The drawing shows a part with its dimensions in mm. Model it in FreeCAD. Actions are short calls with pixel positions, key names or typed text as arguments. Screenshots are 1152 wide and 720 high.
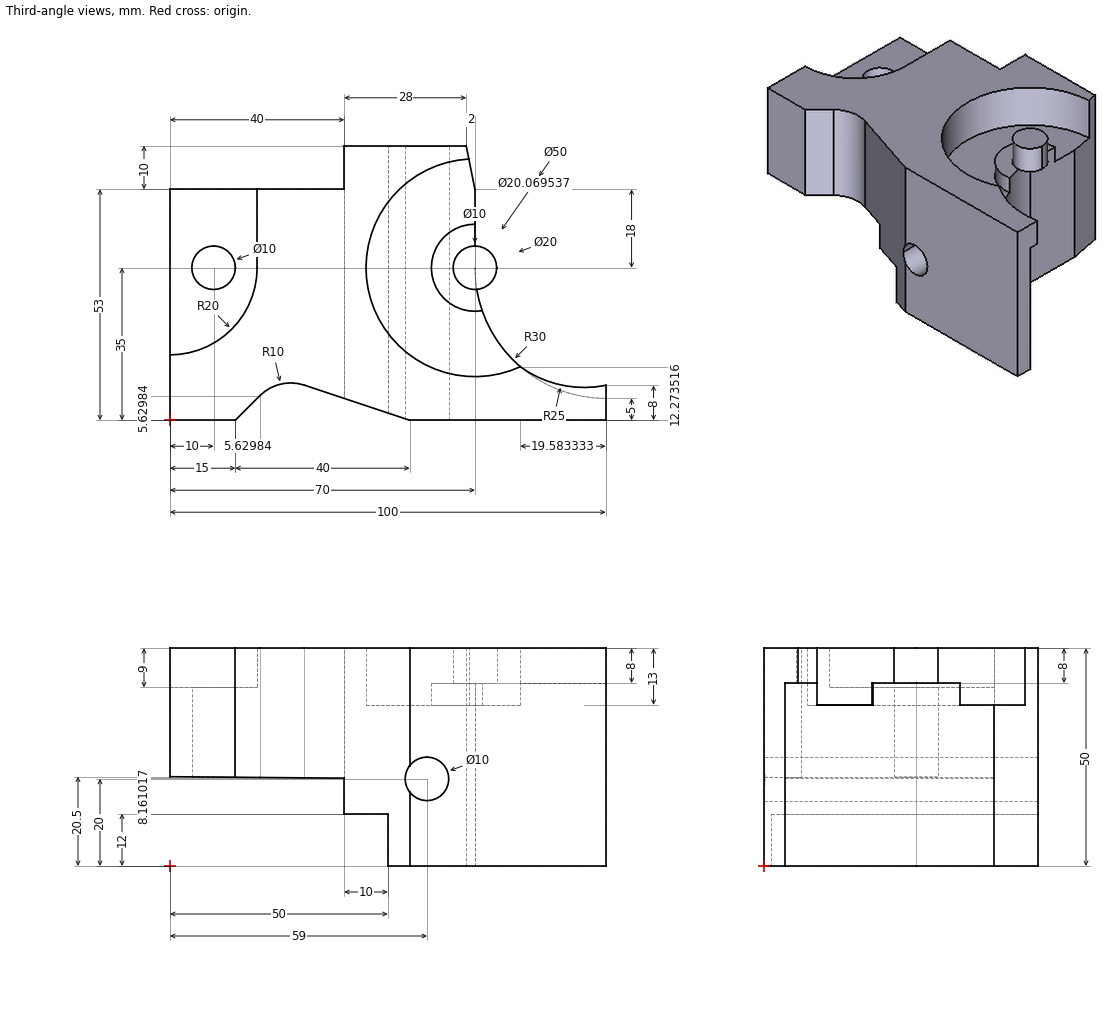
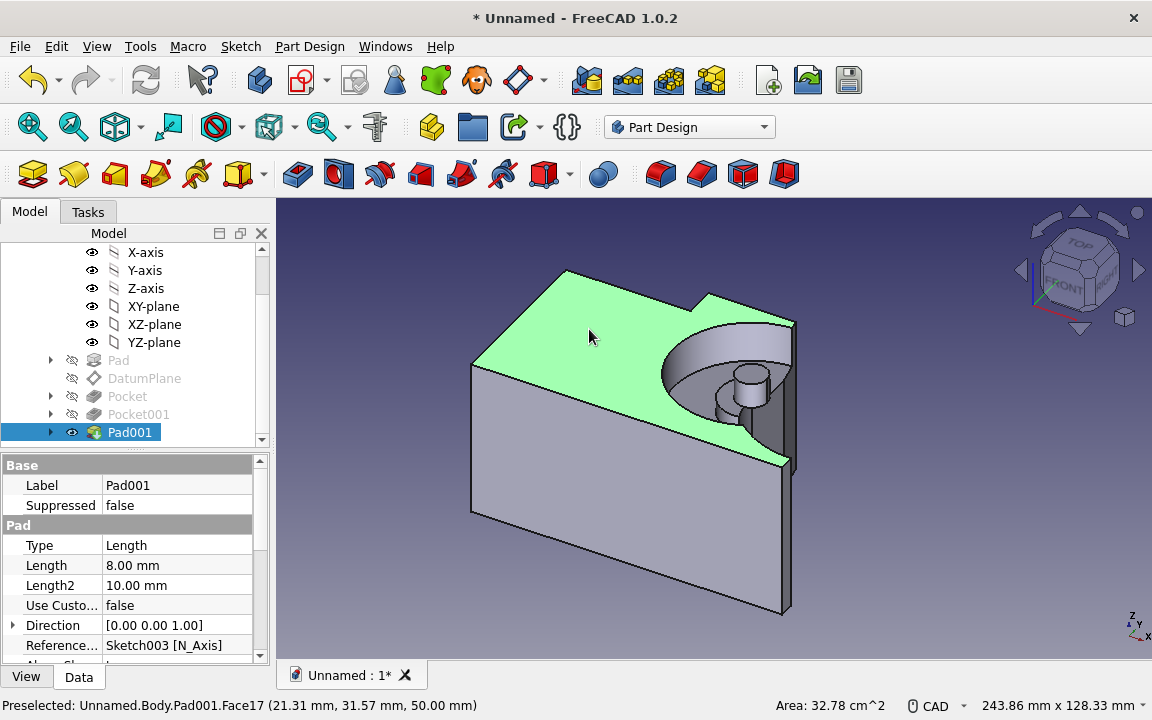
click(300, 80)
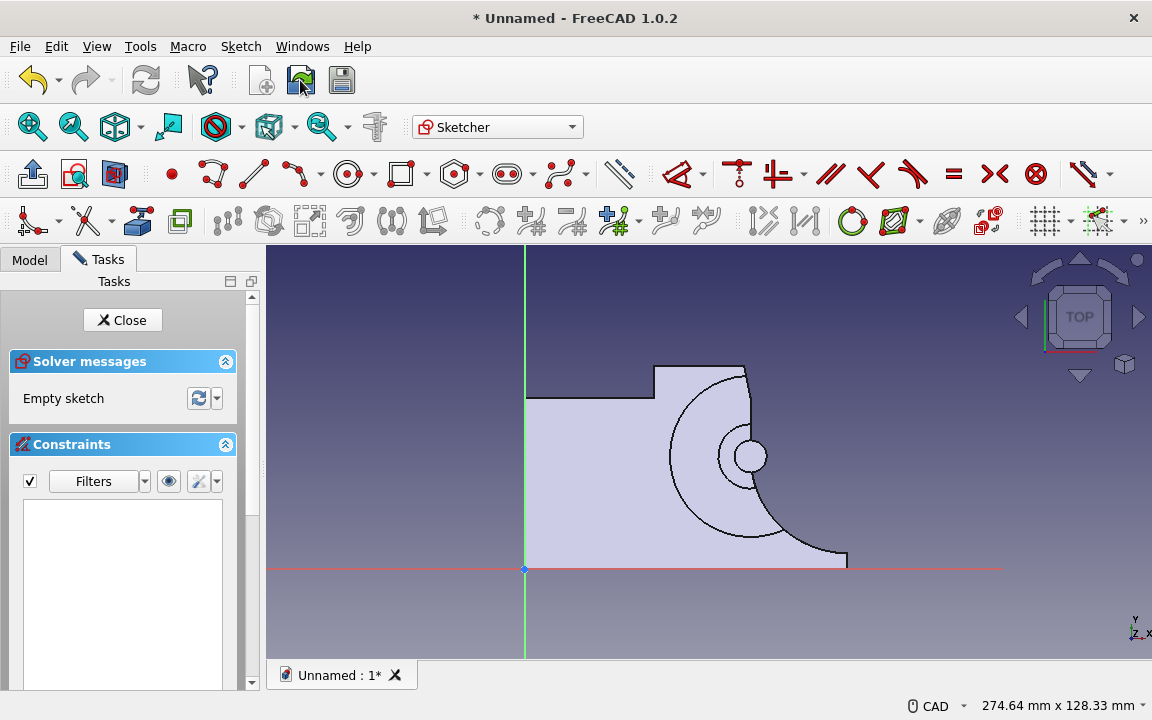
scroll(851, 569, up, 9)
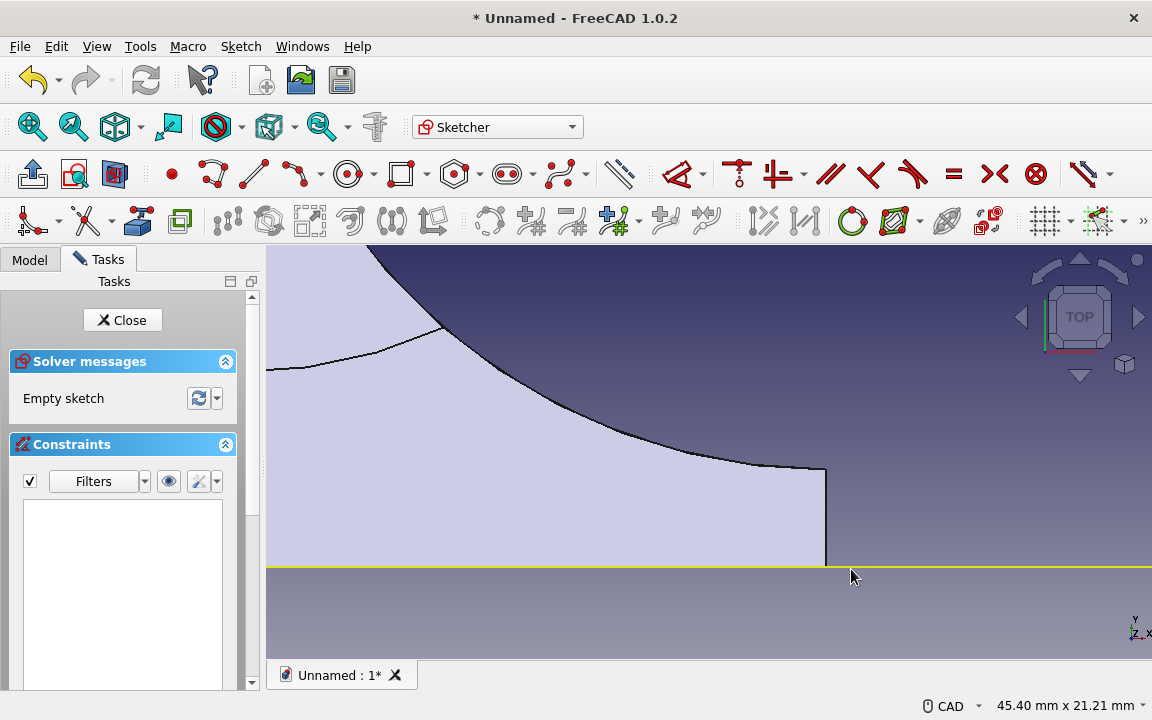
click(213, 174)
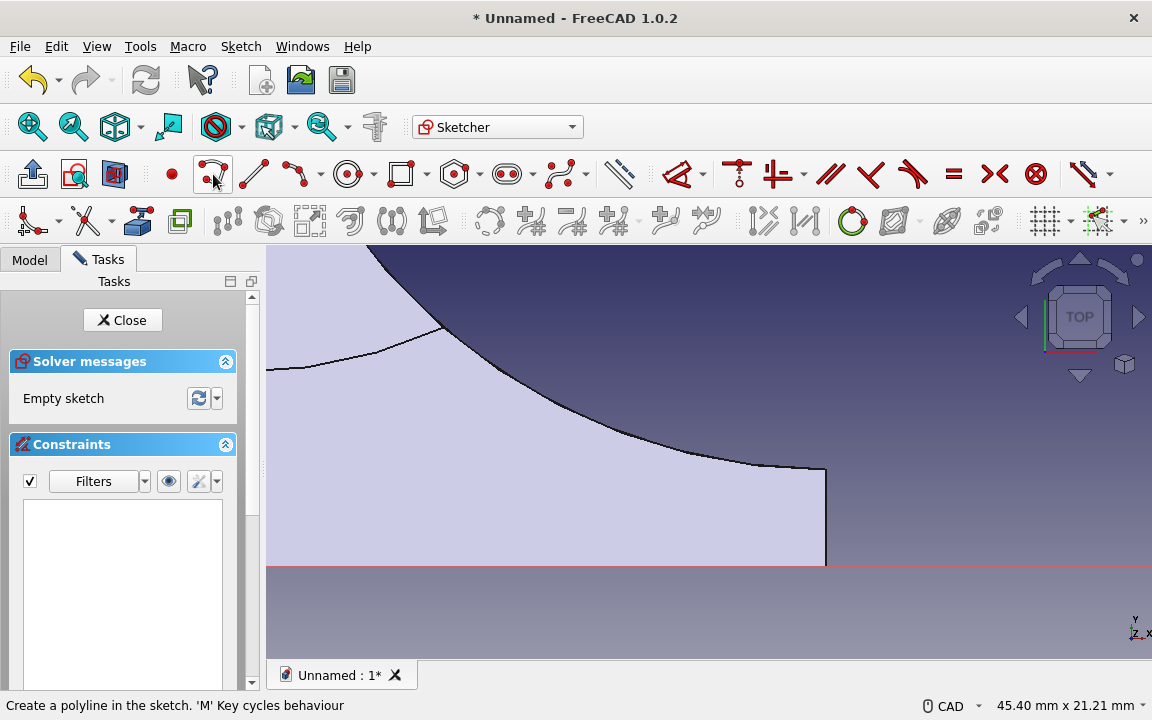
click(444, 328)
click(444, 567)
click(826, 558)
click(826, 411)
right_click(826, 411)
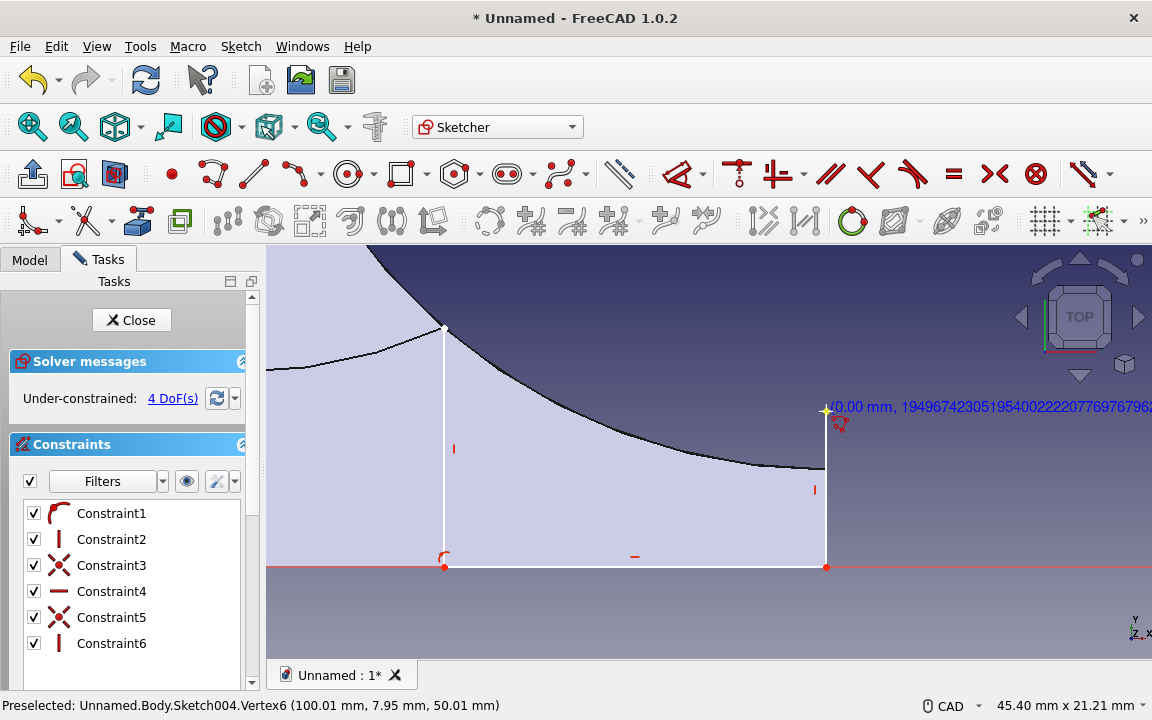
click(294, 174)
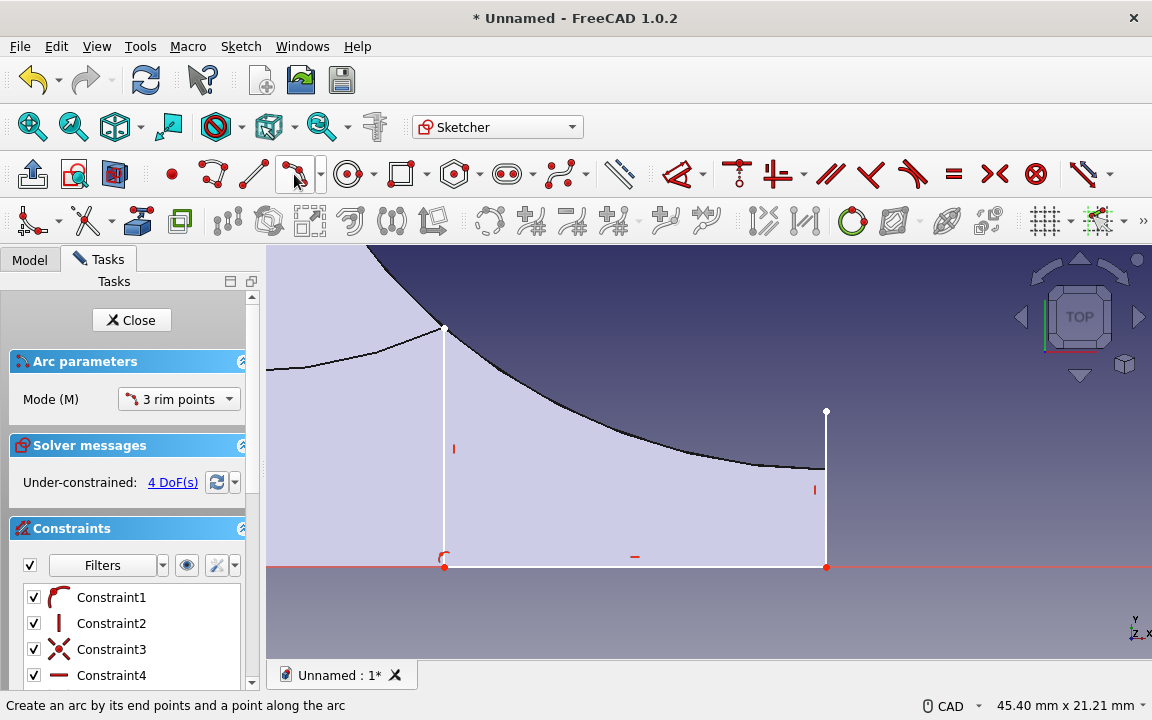
click(826, 412)
click(444, 329)
click(626, 409)
key(Escape)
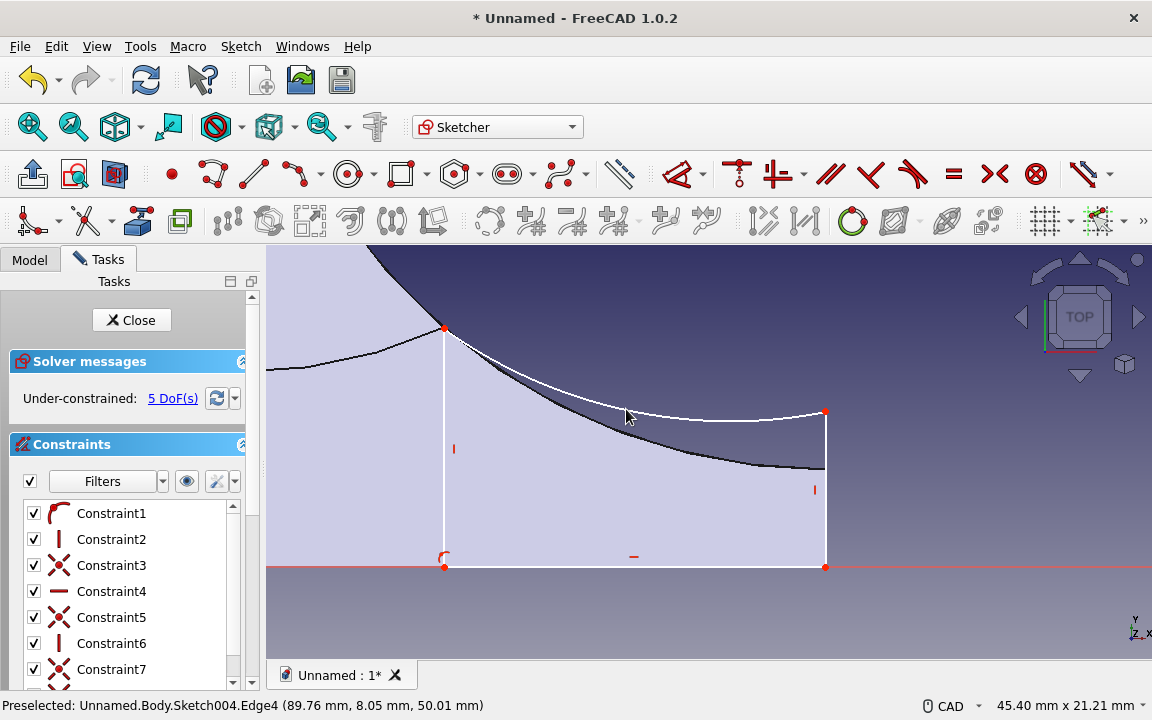
click(676, 174)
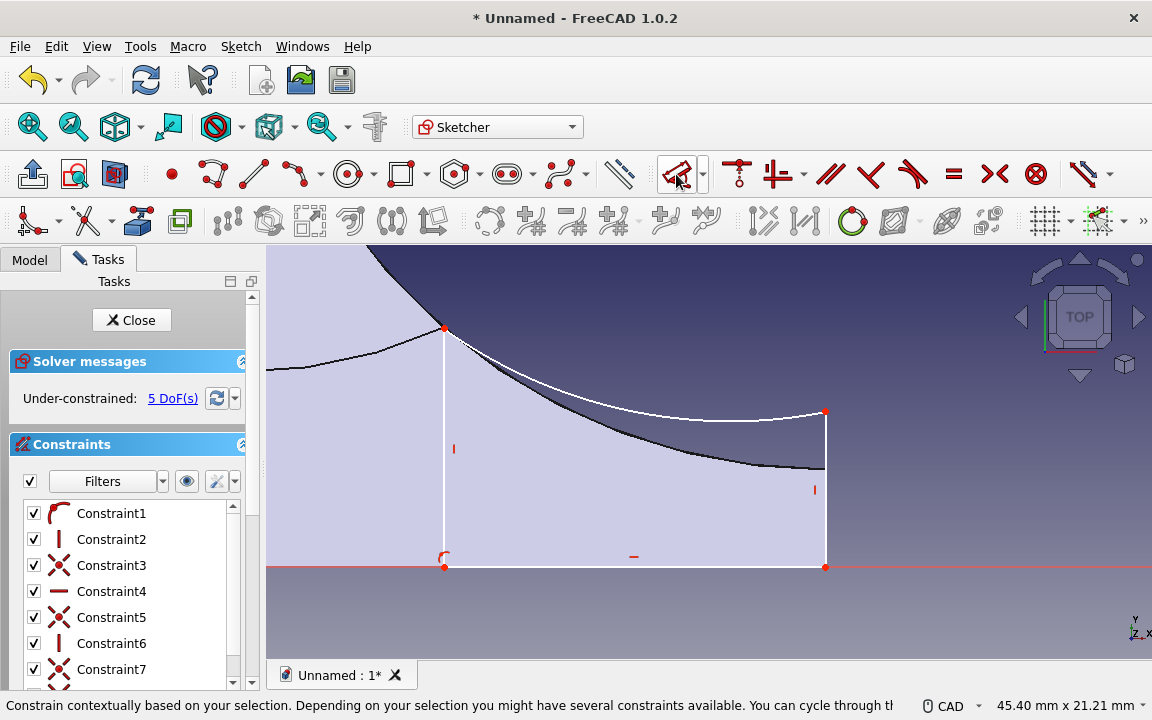
click(550, 387)
click(538, 417)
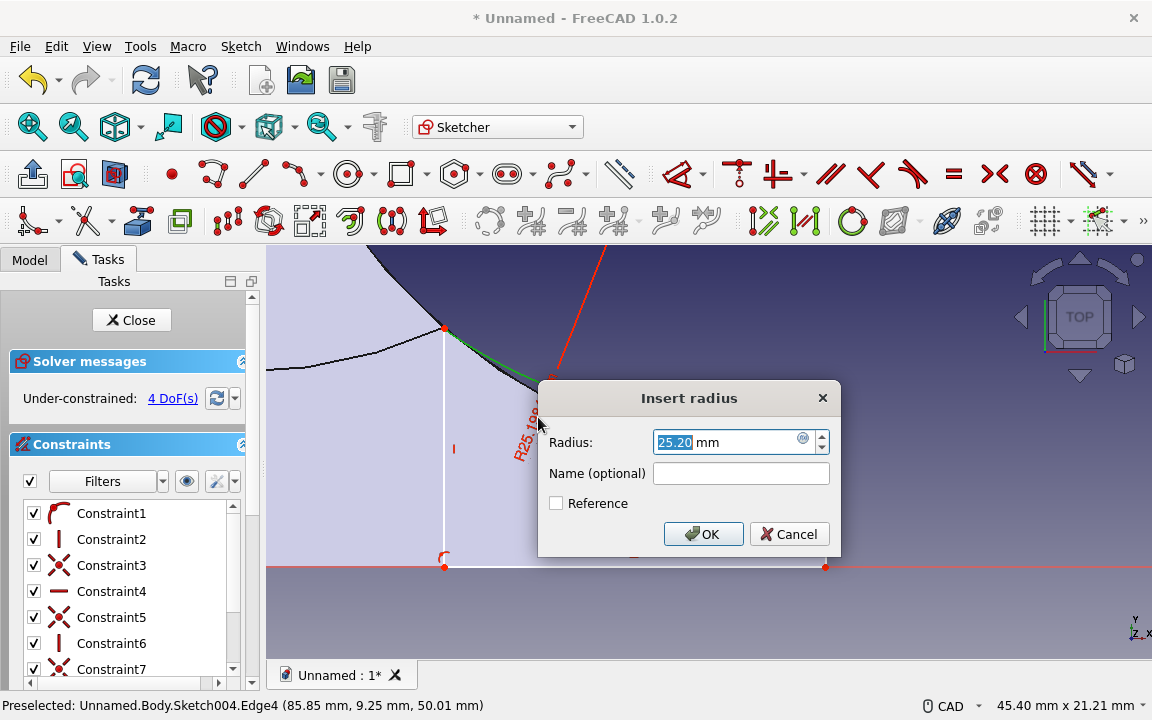
text(25)
key(Return)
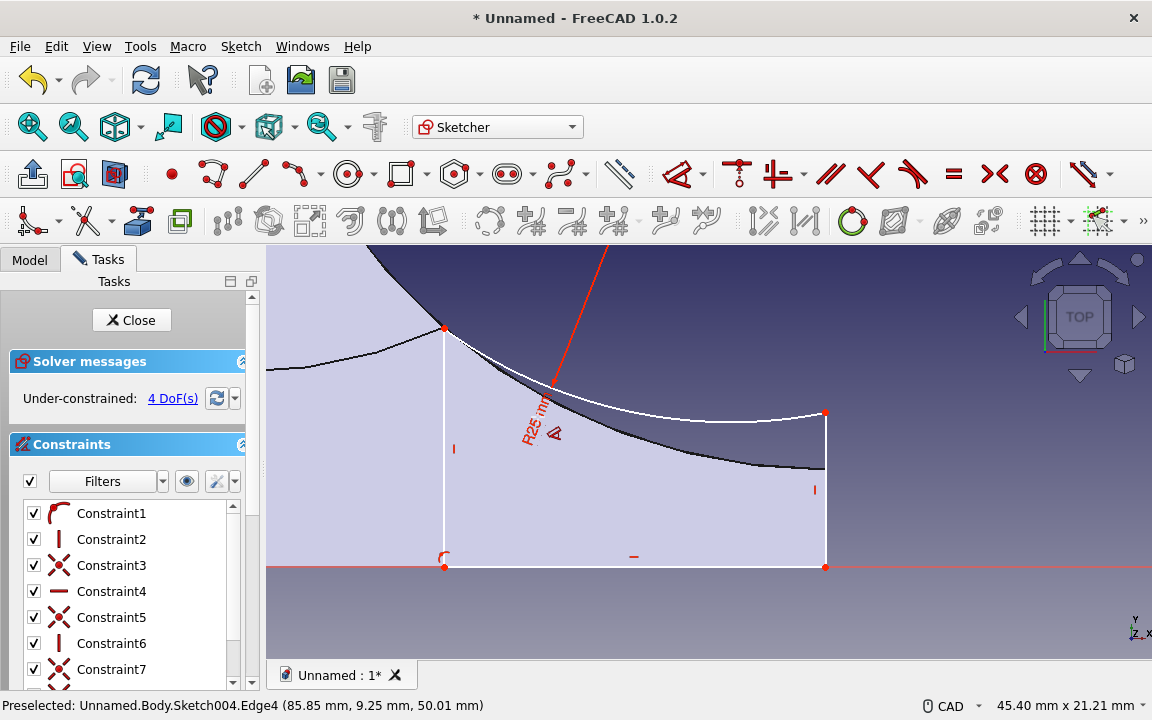
click(826, 521)
click(860, 490)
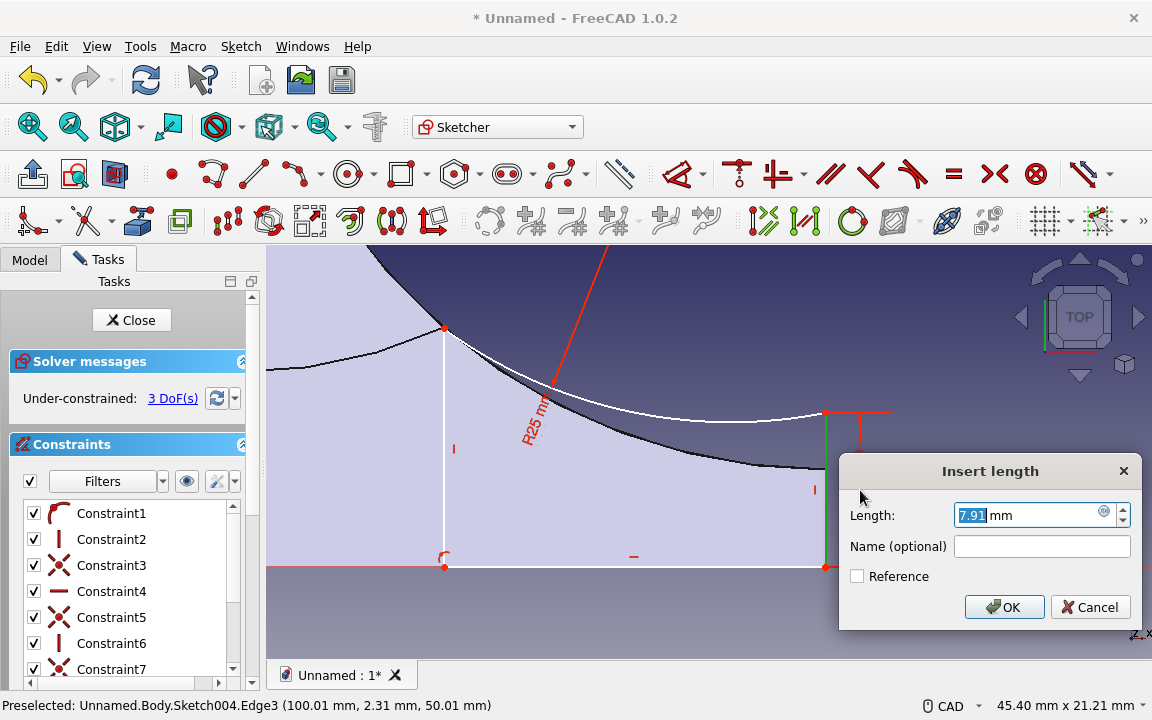
text(8)
key(Return)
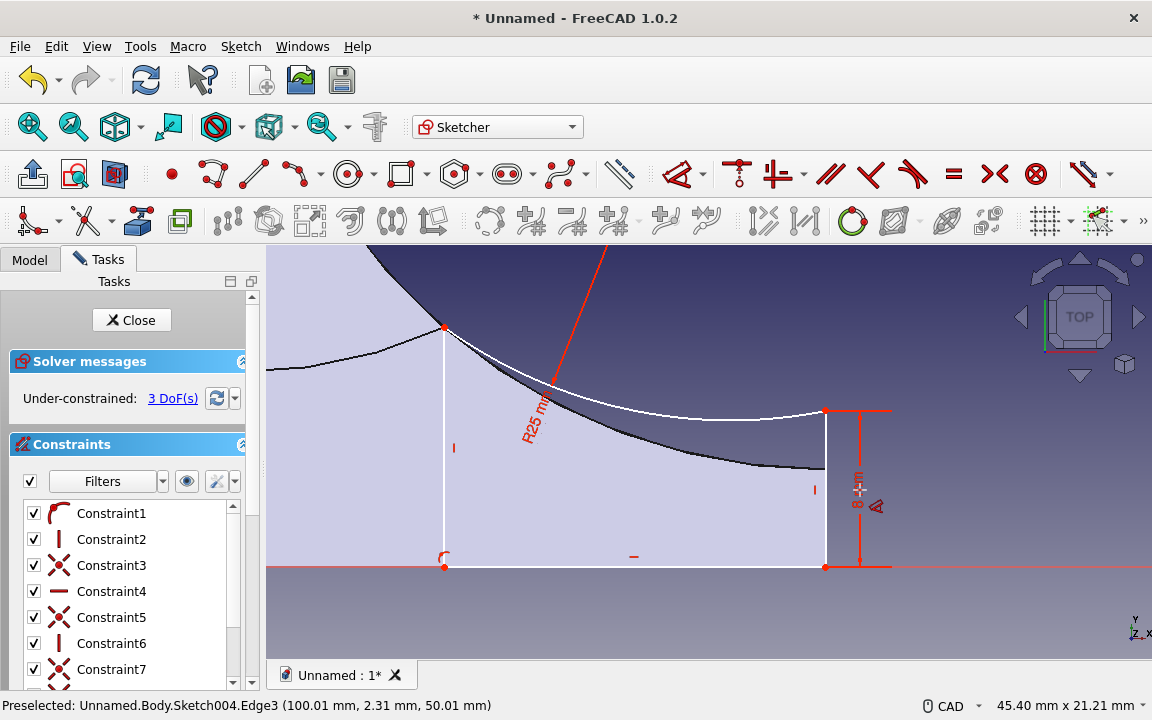
click(826, 567)
click(560, 601)